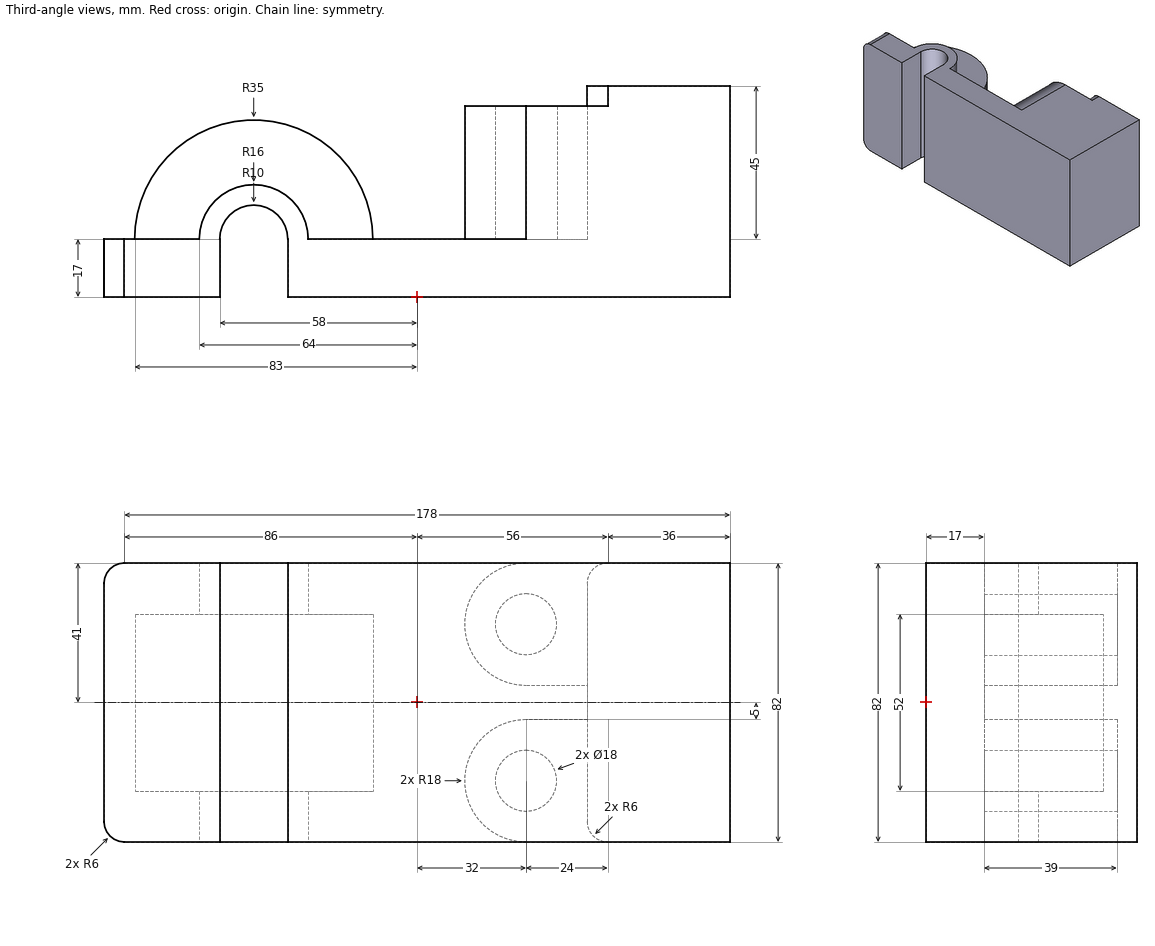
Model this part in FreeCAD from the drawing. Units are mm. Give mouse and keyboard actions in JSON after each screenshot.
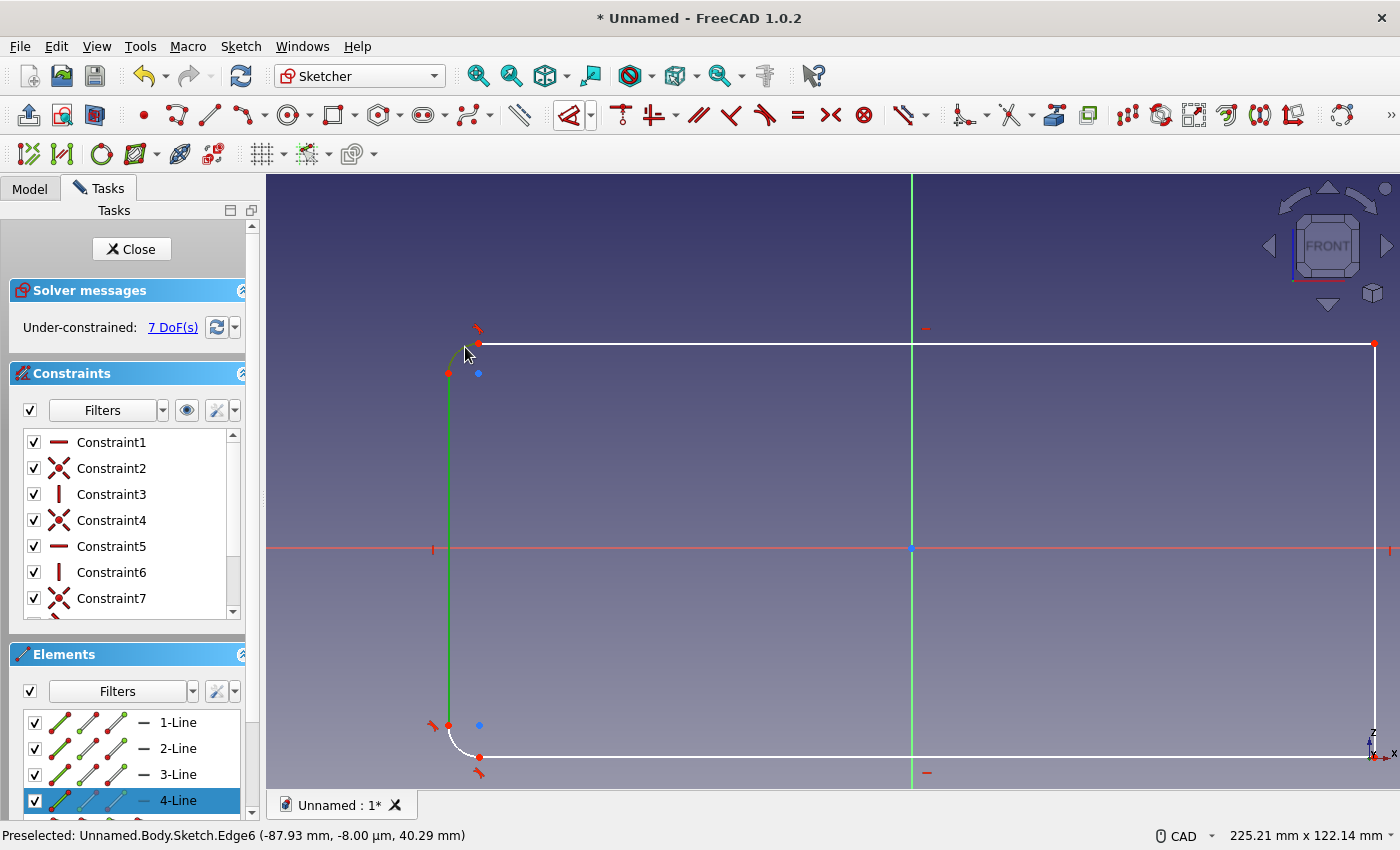
{"action": "left_click", "coordinate": [765, 116]}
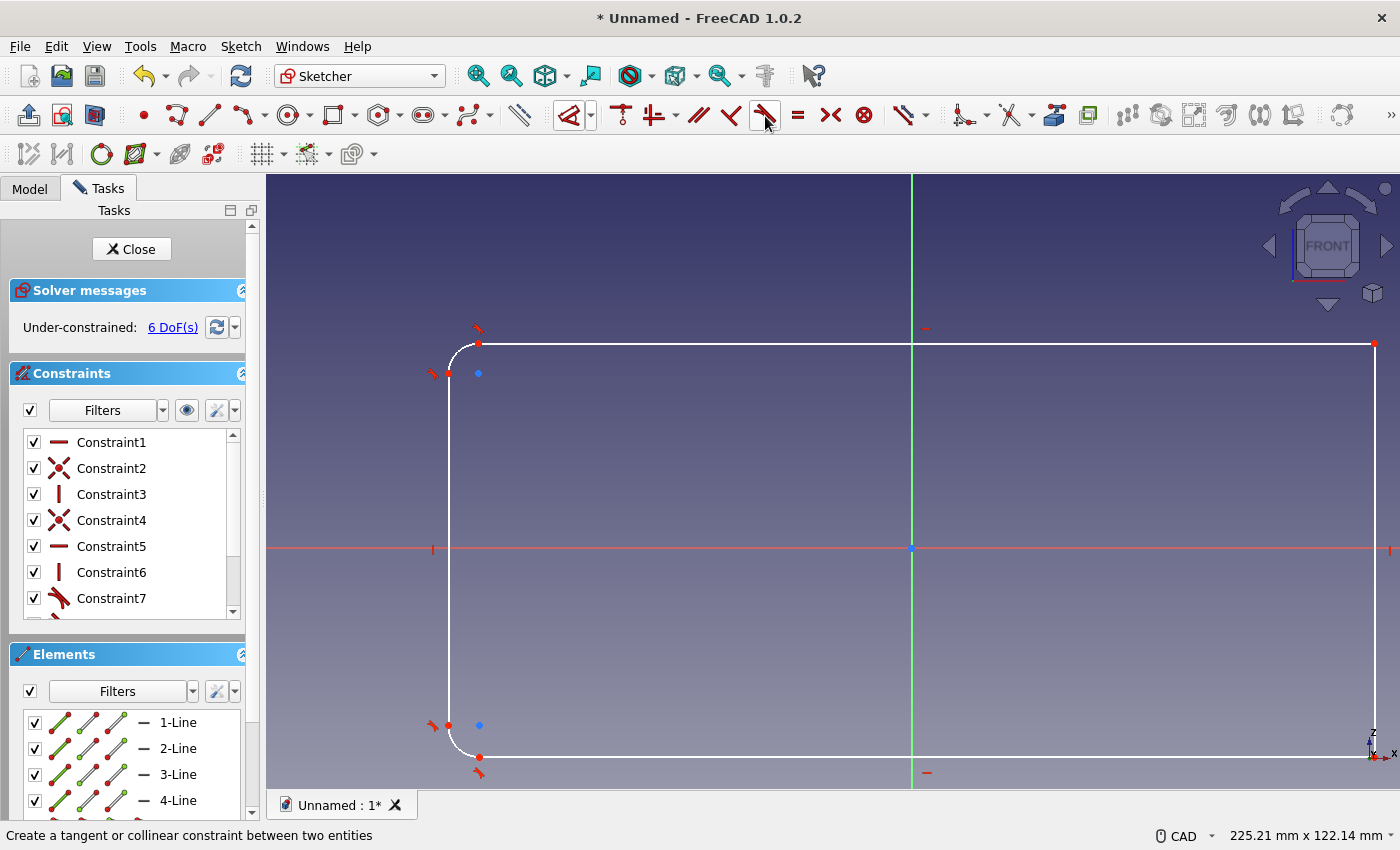
{"action": "left_click", "coordinate": [452, 740]}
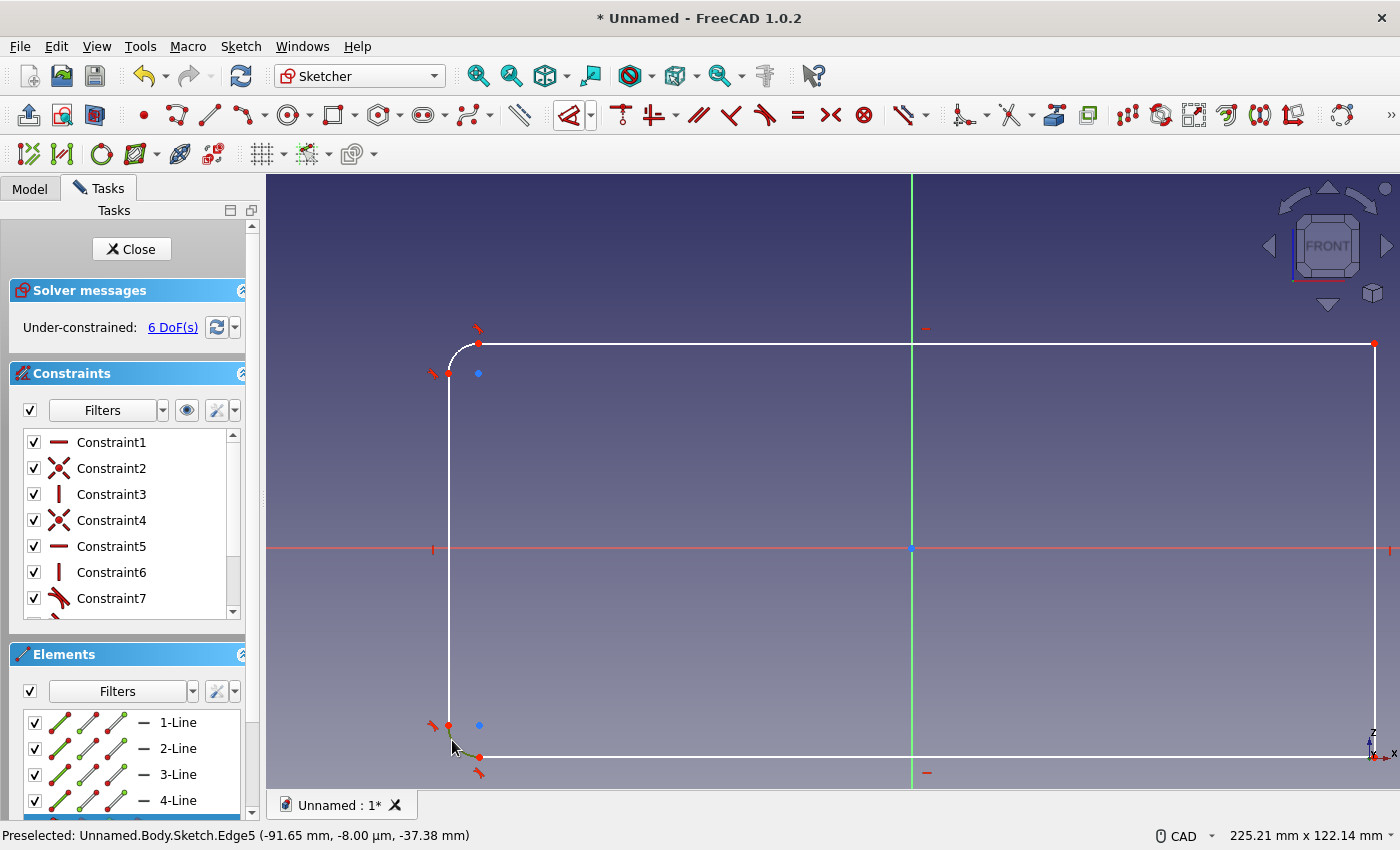
{"action": "left_click", "coordinate": [465, 347]}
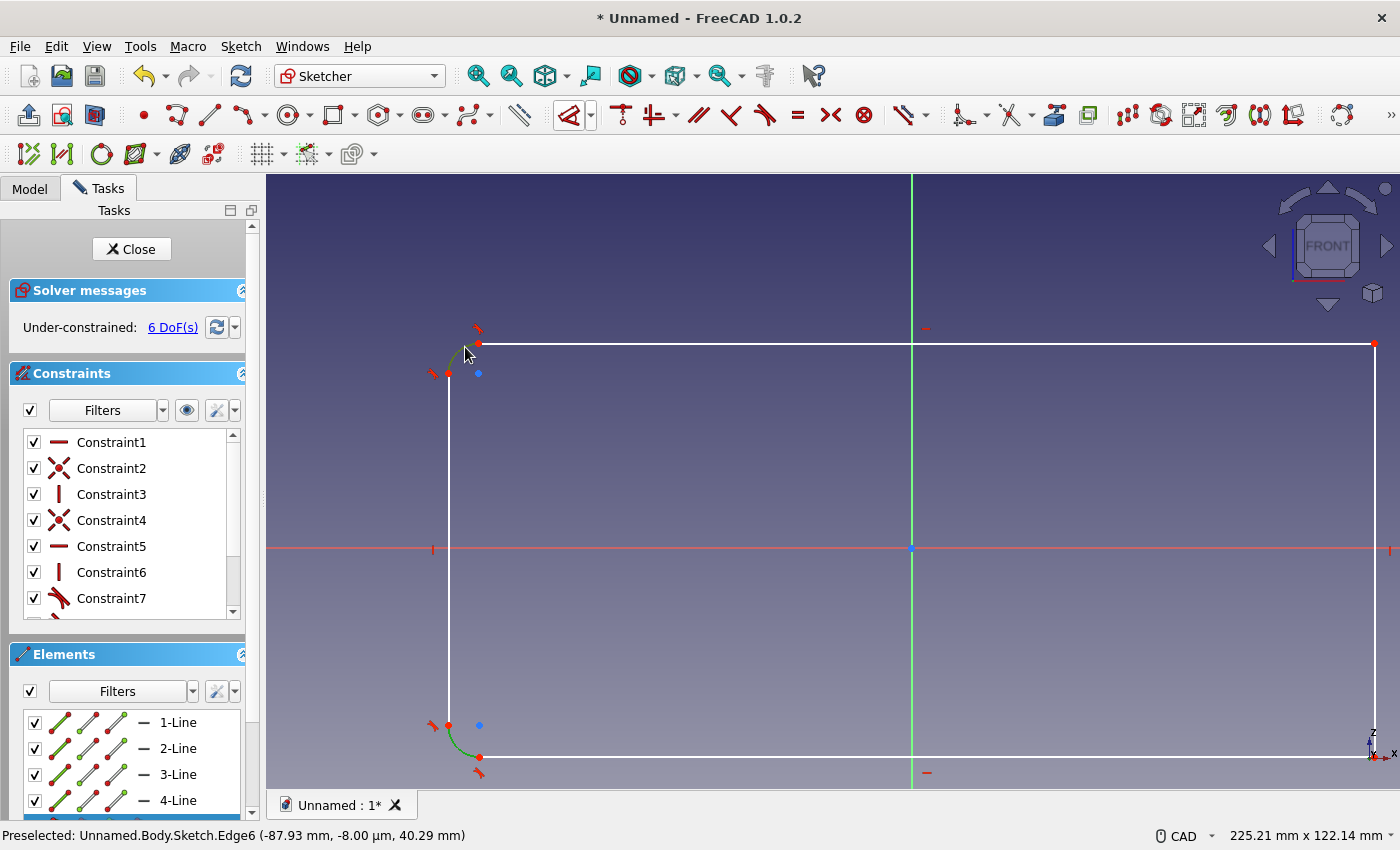
{"action": "left_click", "coordinate": [798, 116]}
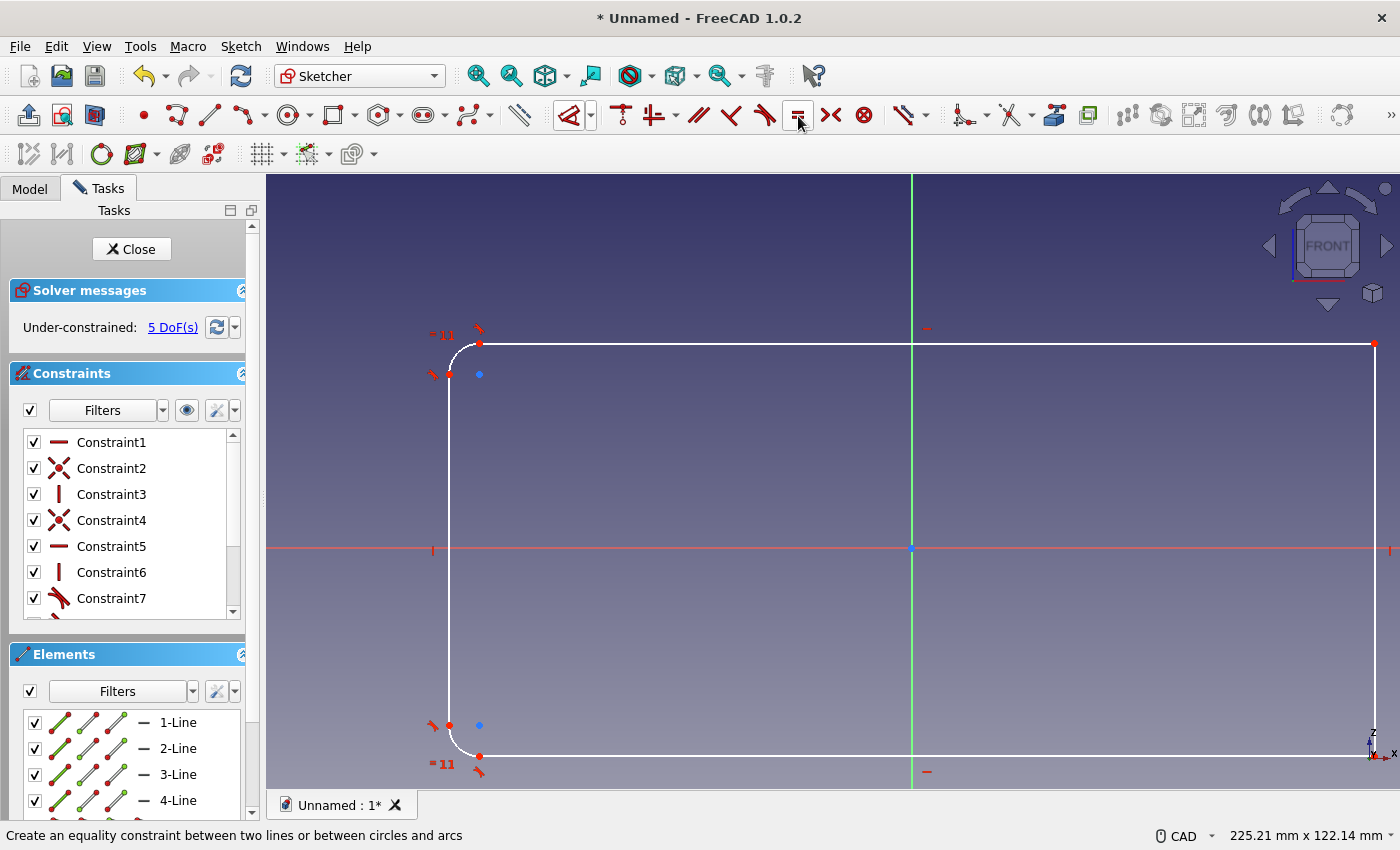
{"action": "scroll", "coordinate": [453, 740], "scroll_direction": "up", "scroll_amount": 2}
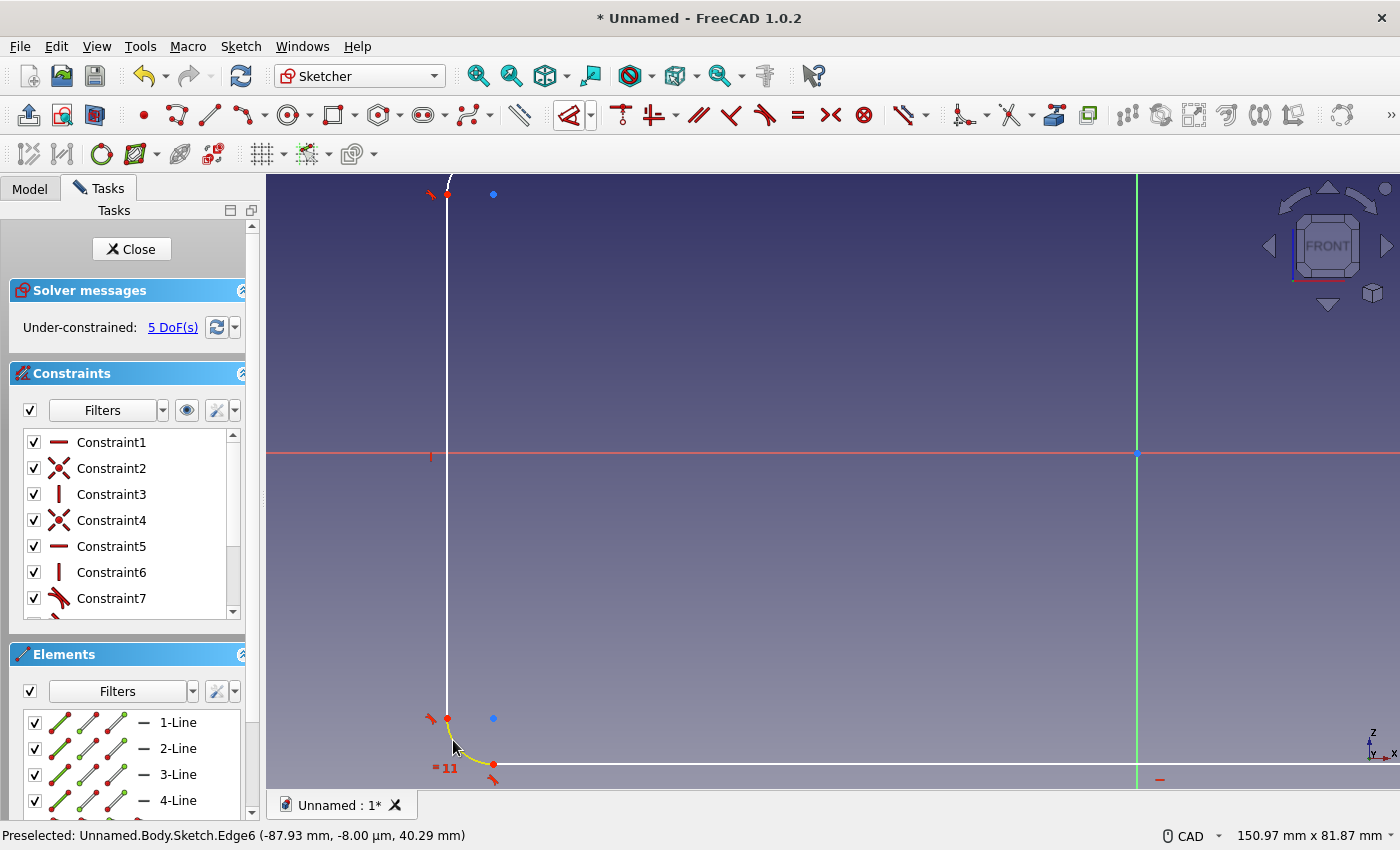
{"action": "left_click", "coordinate": [452, 739]}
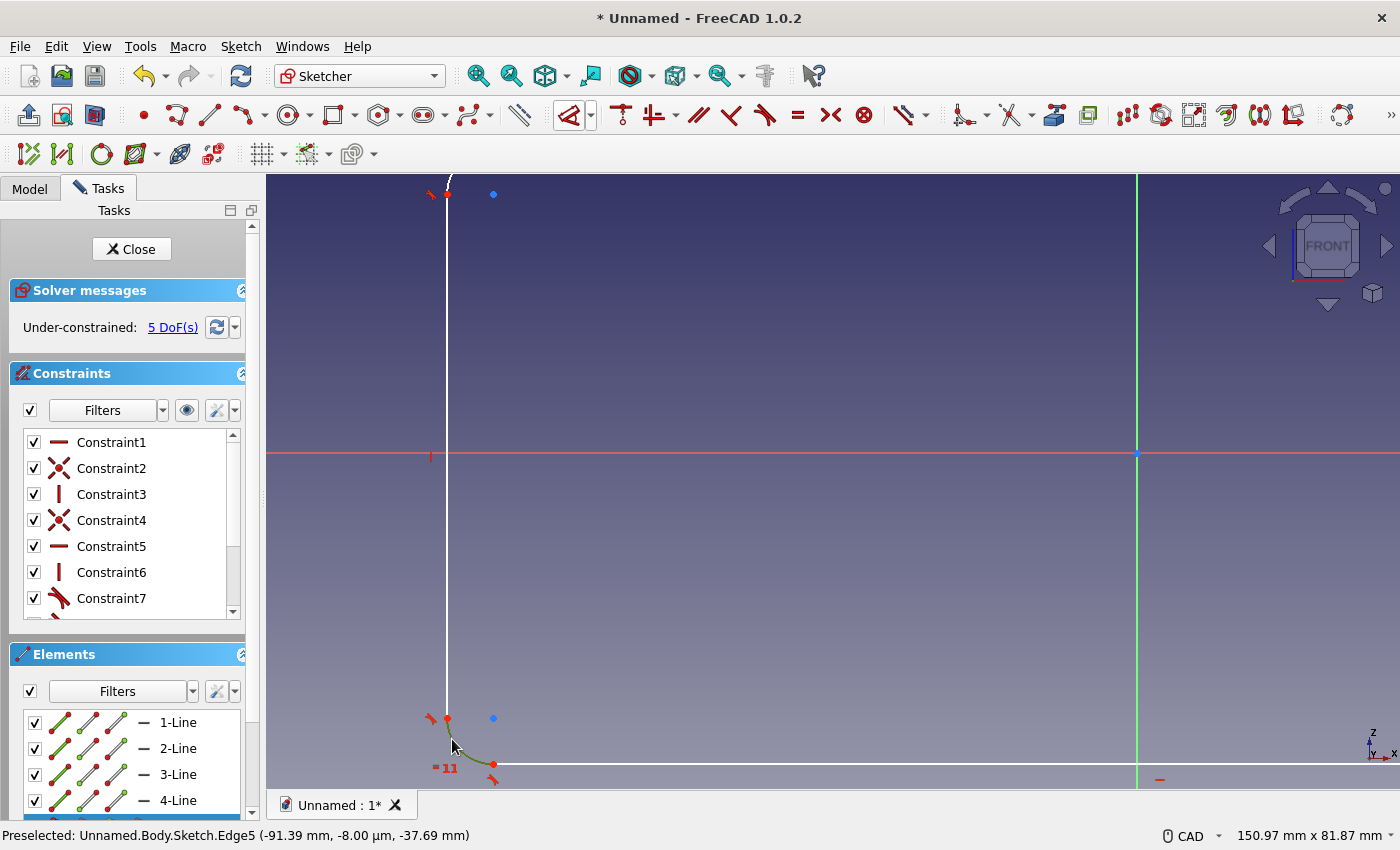
{"action": "left_click", "coordinate": [590, 116]}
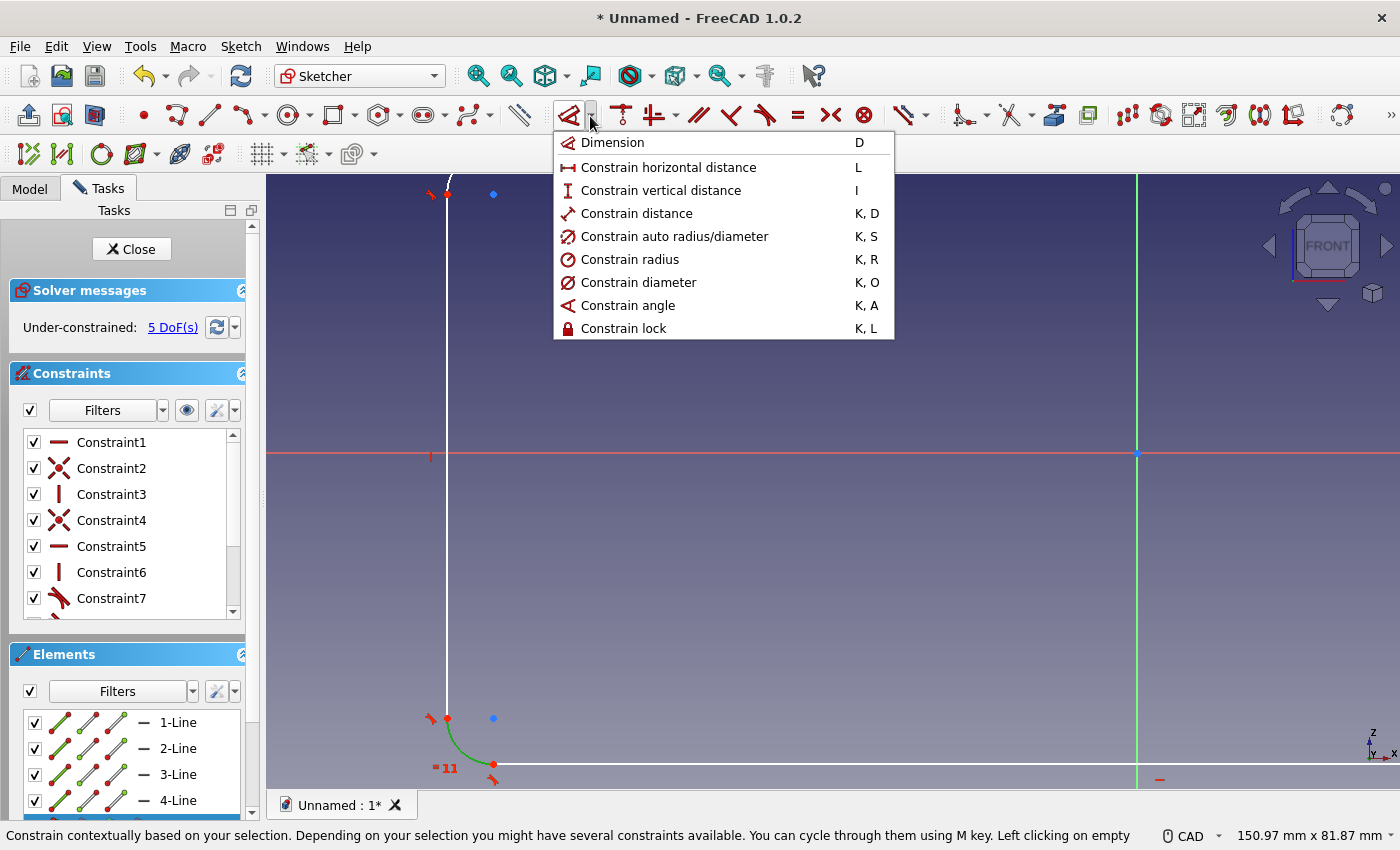
{"action": "left_click", "coordinate": [724, 260]}